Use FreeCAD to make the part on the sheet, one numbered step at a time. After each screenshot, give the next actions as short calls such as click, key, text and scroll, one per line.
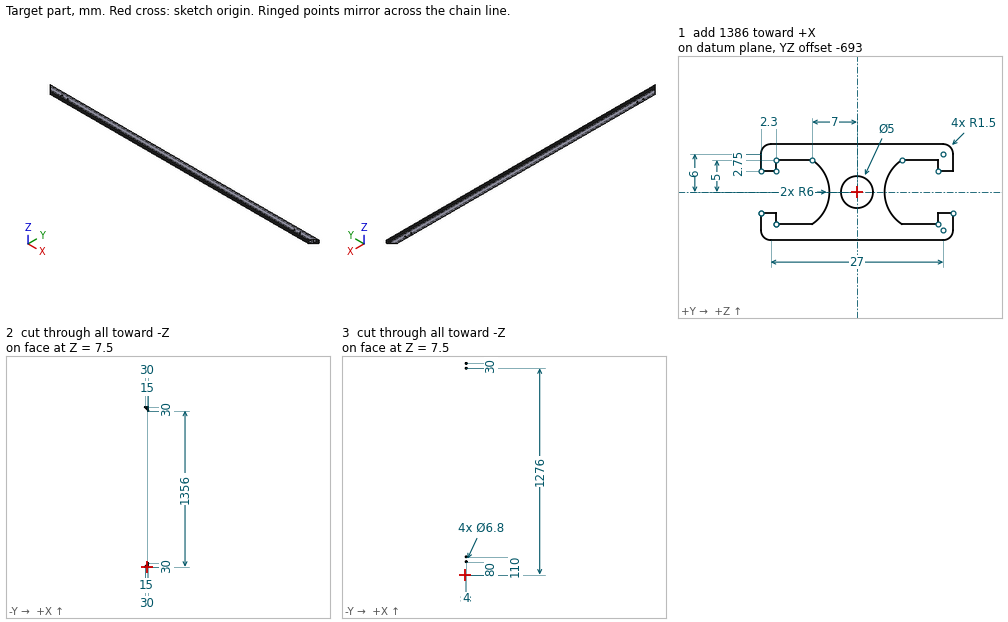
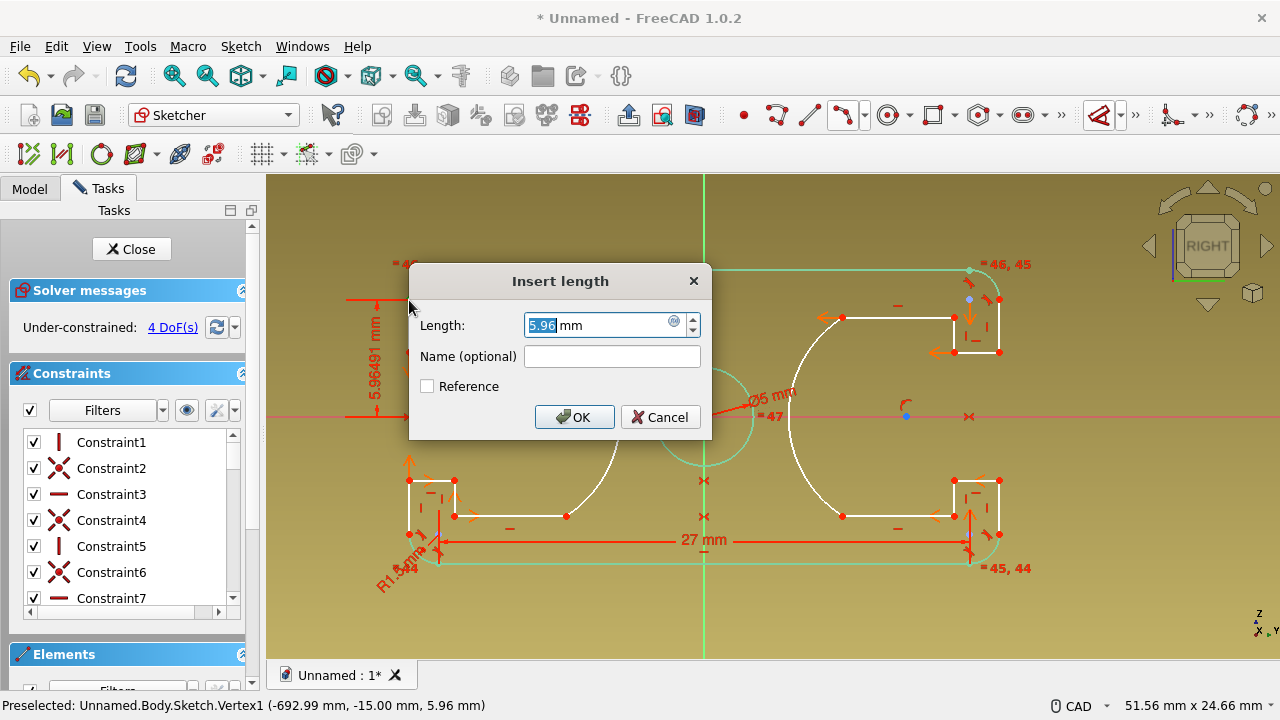
text(6)
key(Return)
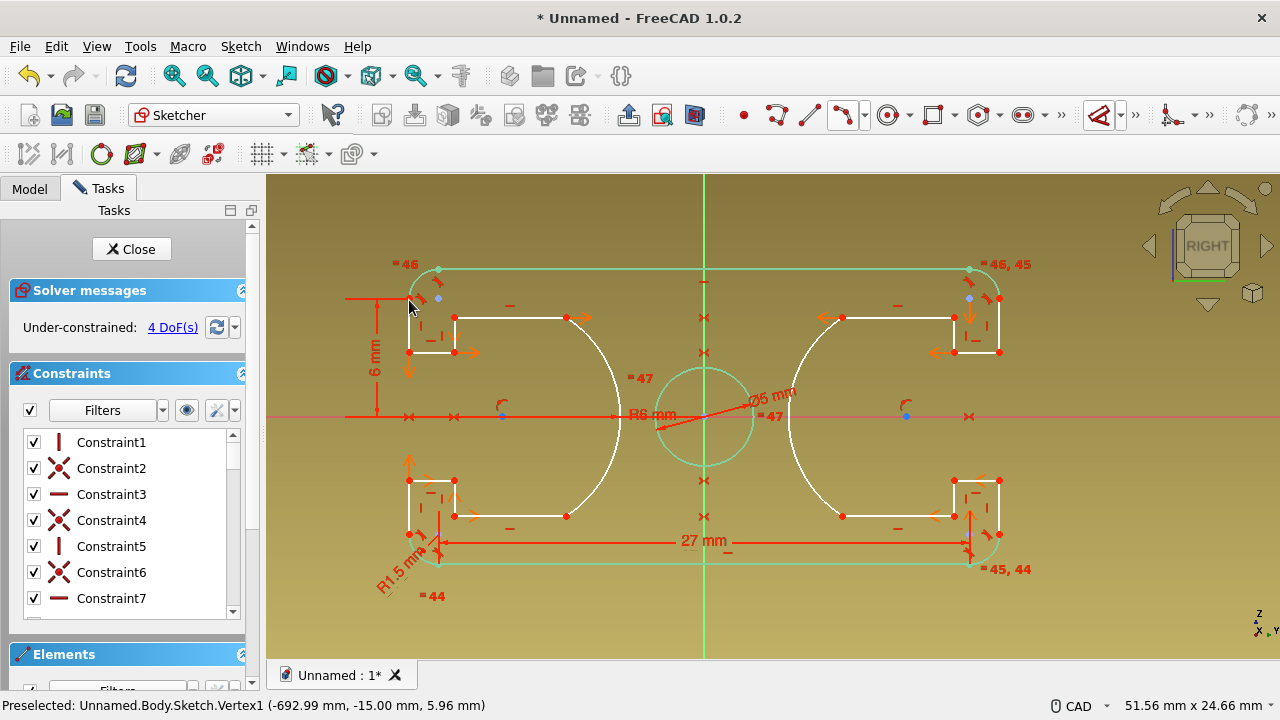
click(455, 318)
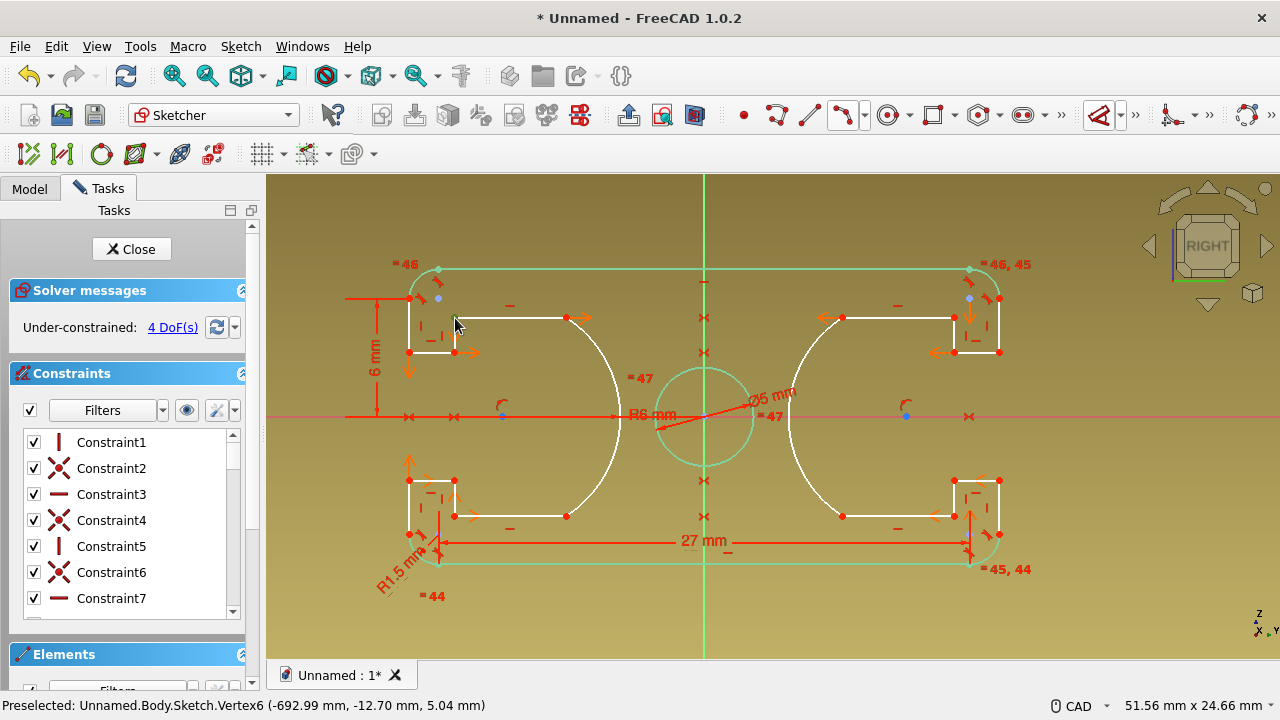
key(i)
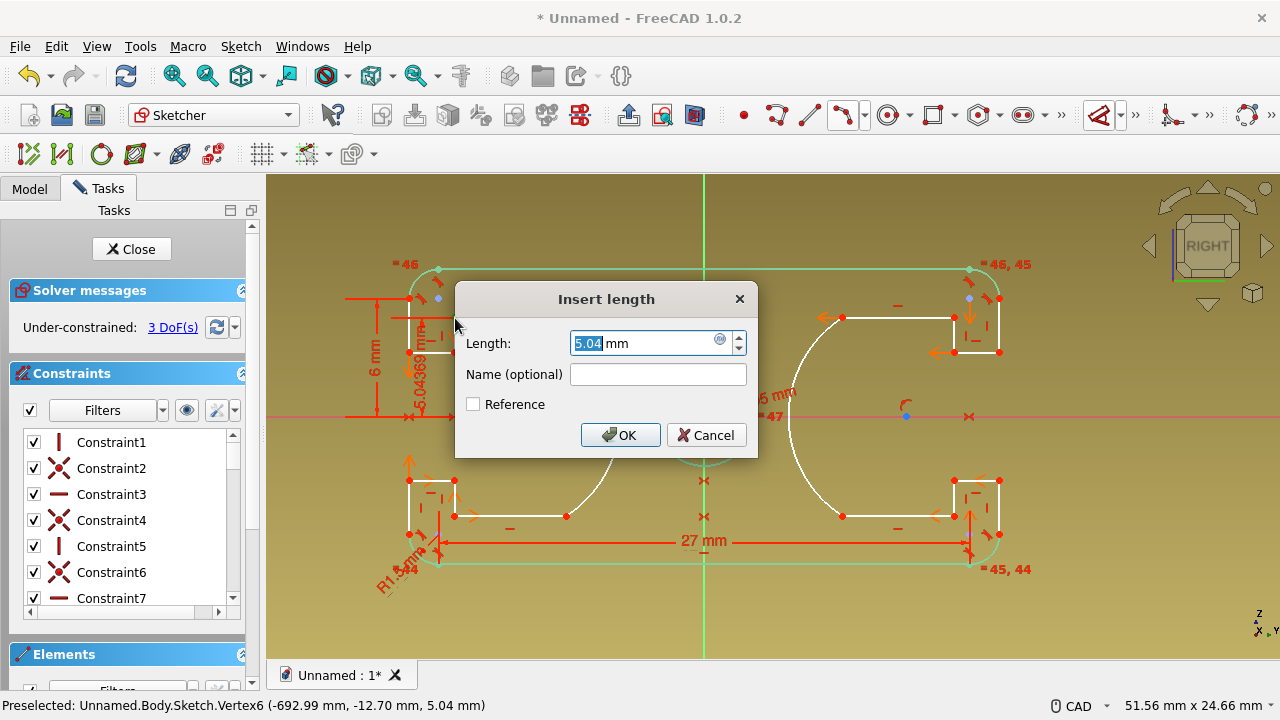
text(5)
key(Return)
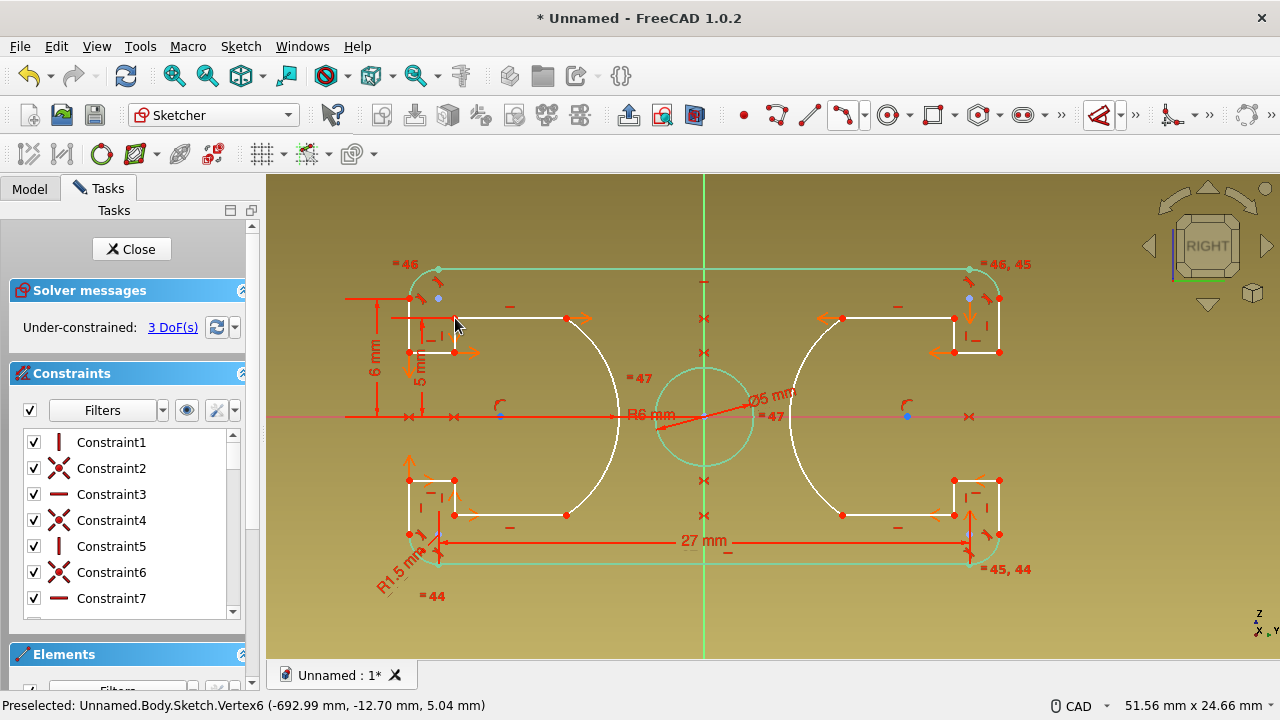
click(566, 318)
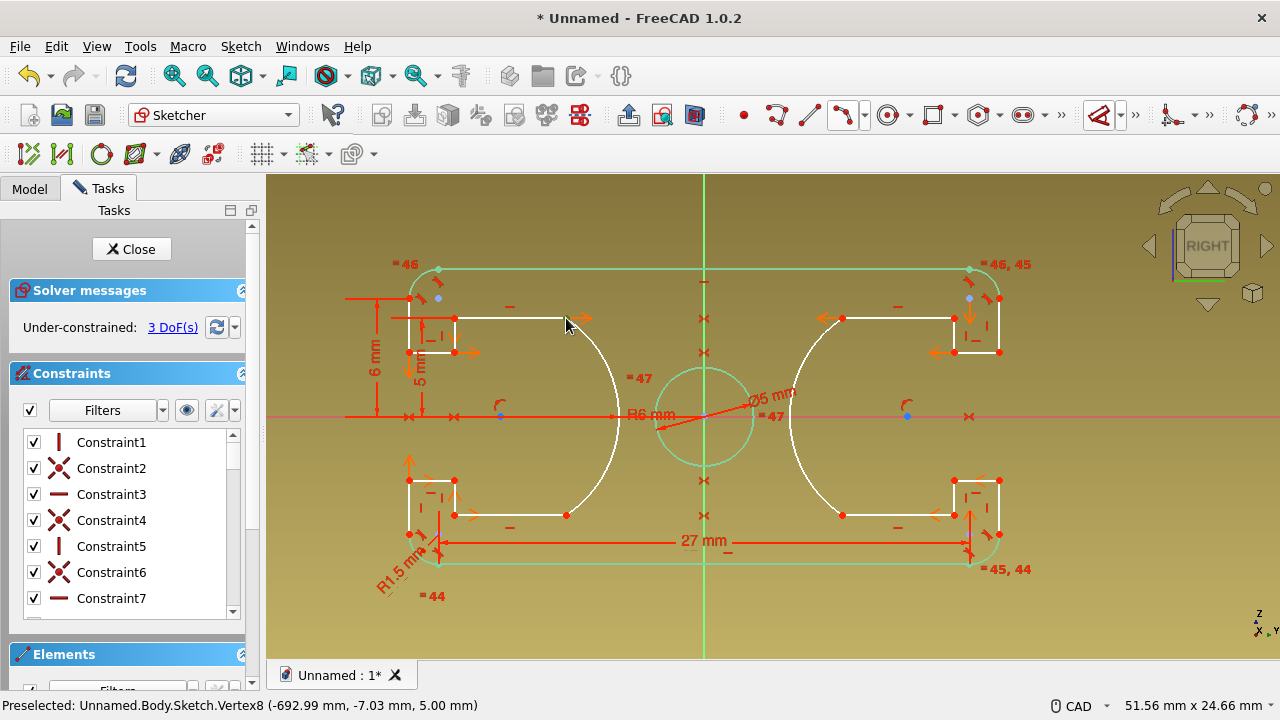
key(l)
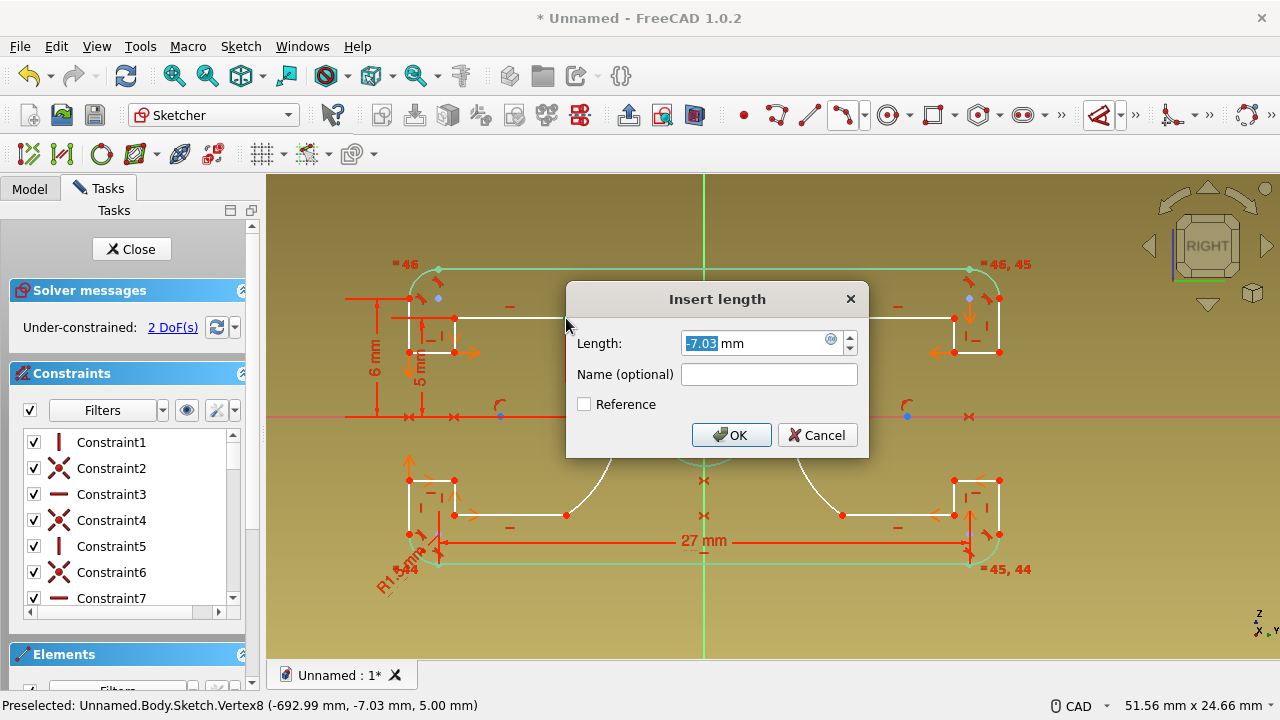
text(-7)
key(Return)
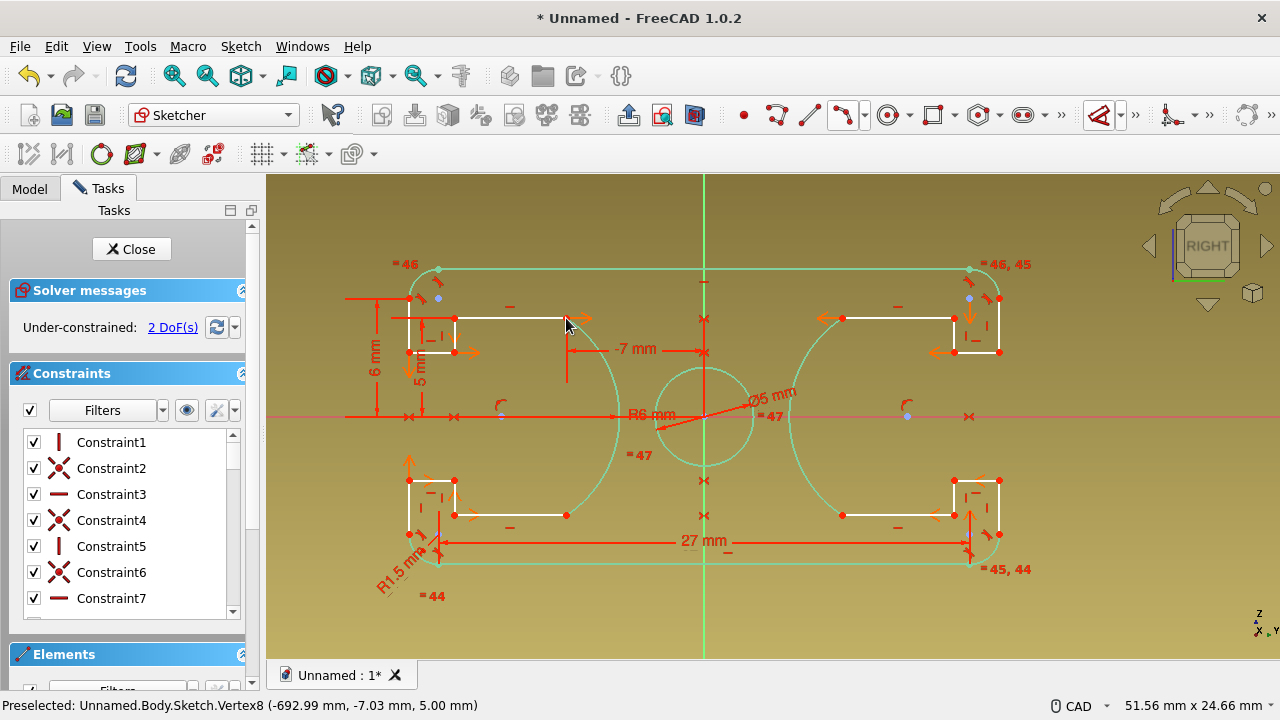
click(441, 353)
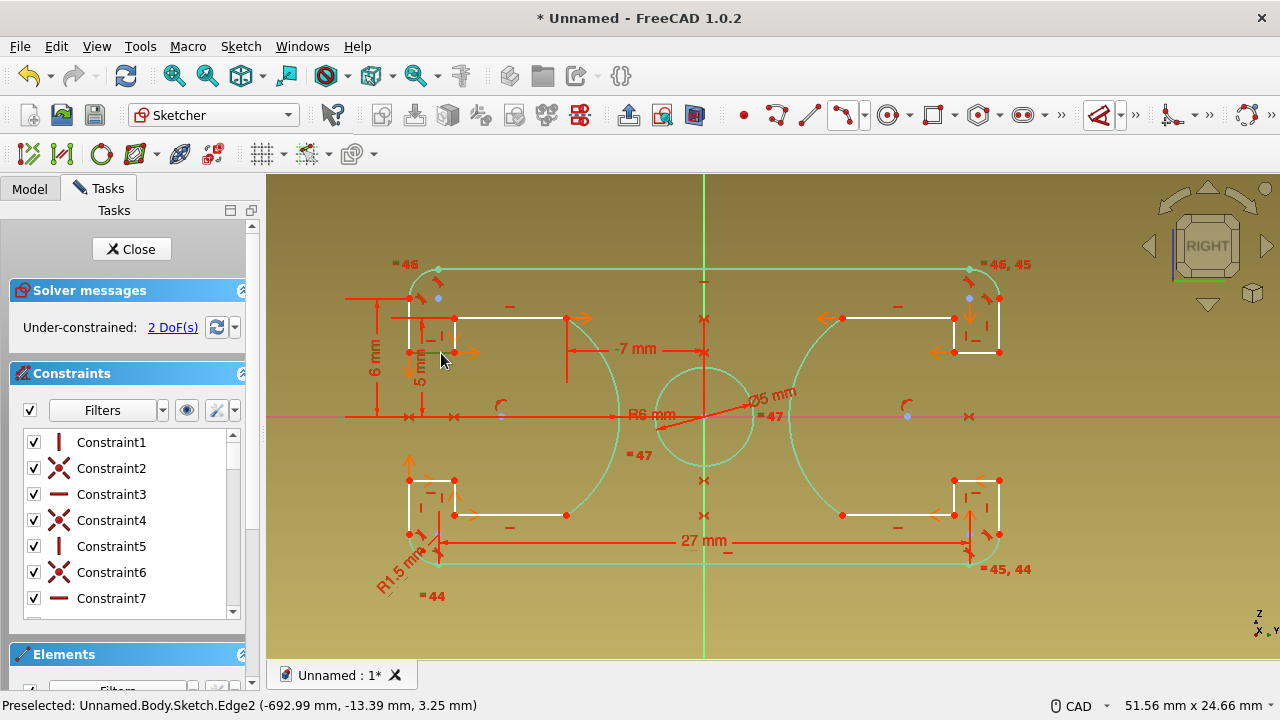
key(l)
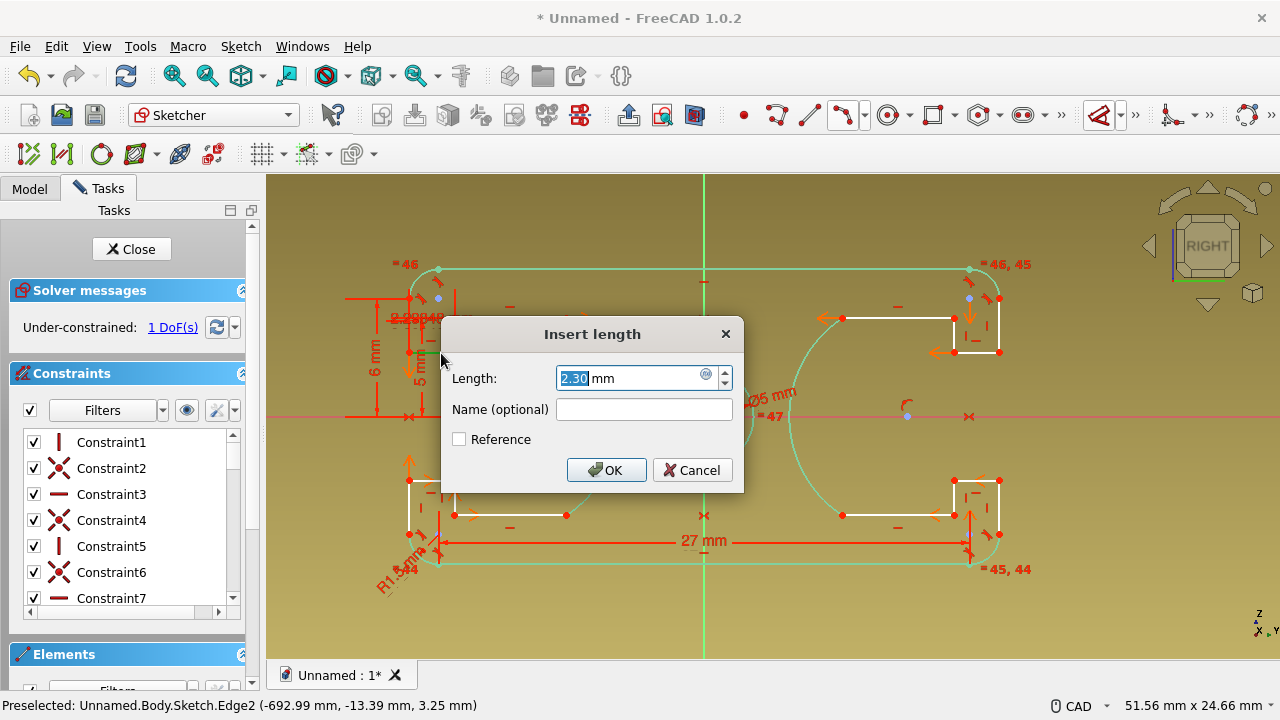
text(2.3)
key(Return)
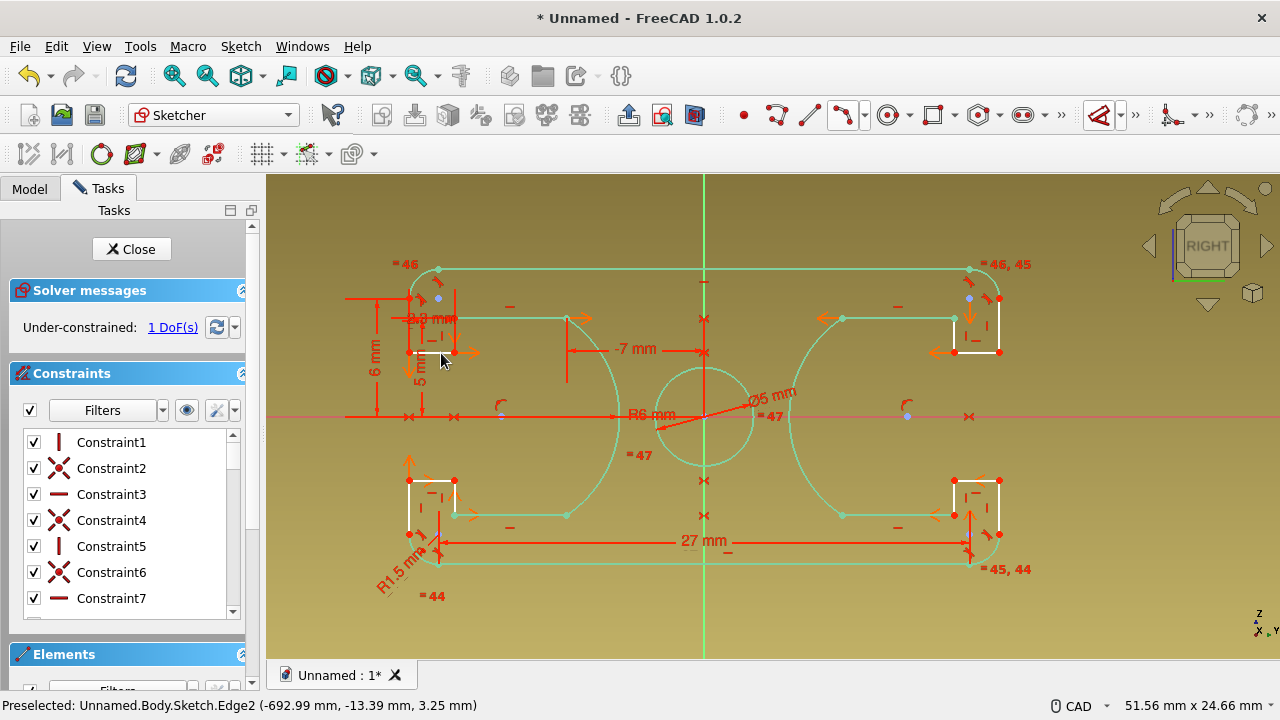
click(409, 337)